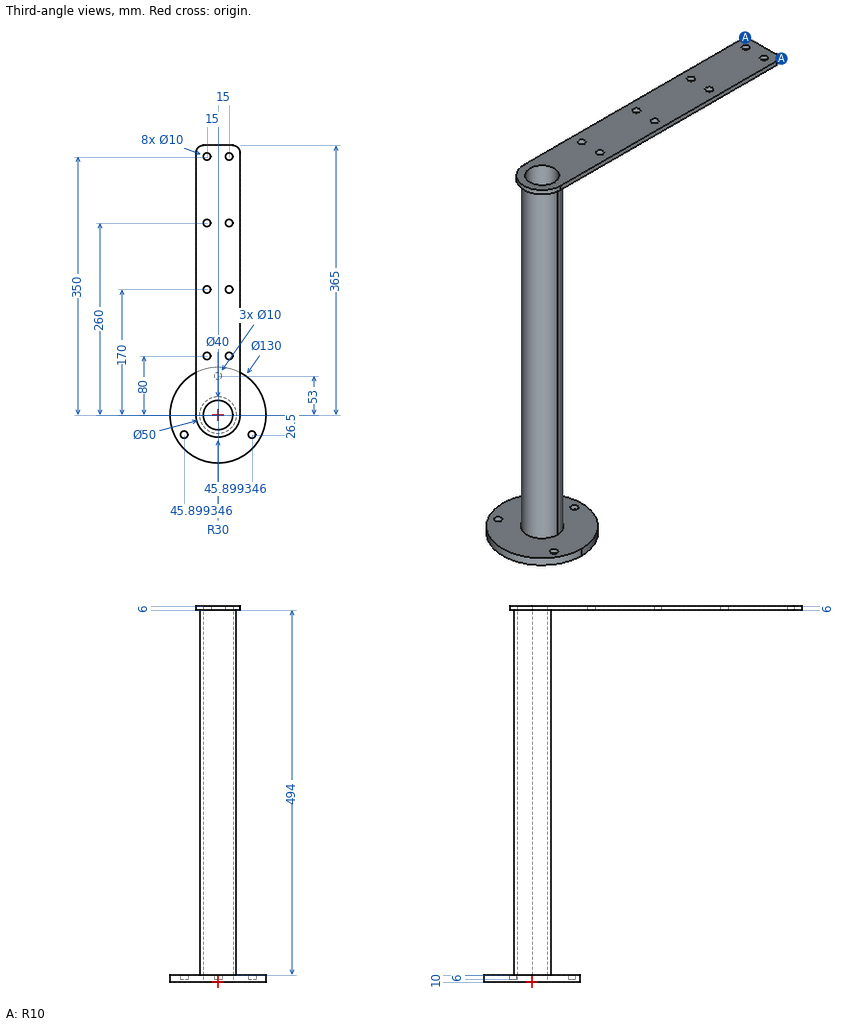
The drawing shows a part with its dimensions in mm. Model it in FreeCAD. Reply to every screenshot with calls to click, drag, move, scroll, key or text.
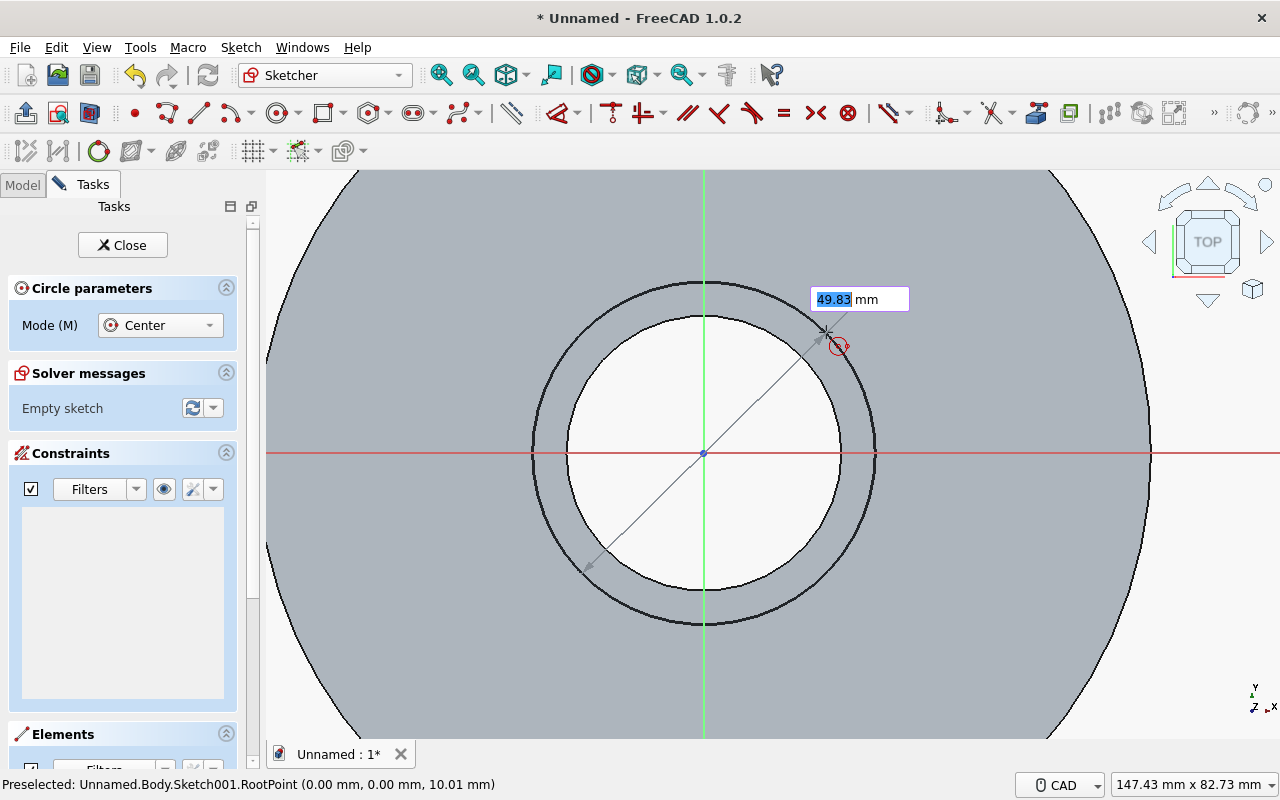
text(50)
key(Return)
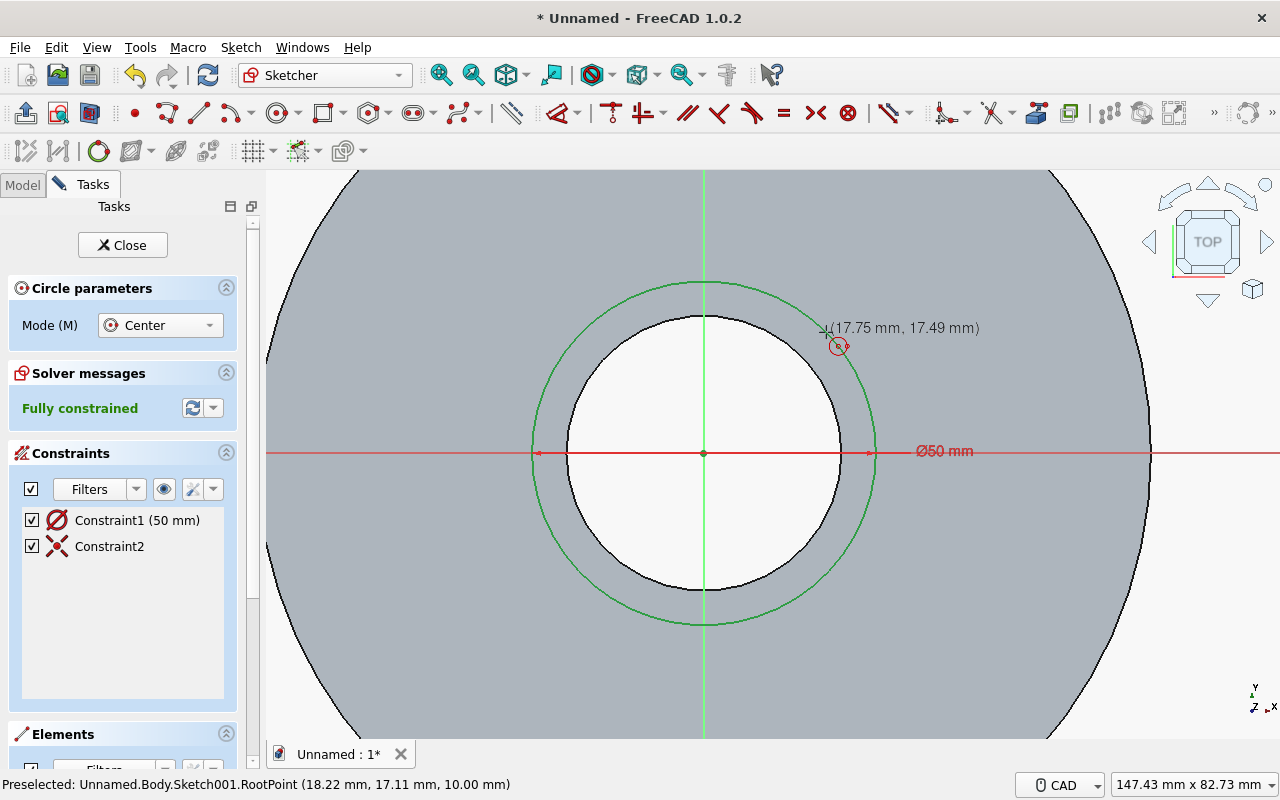
click(704, 453)
move(801, 356)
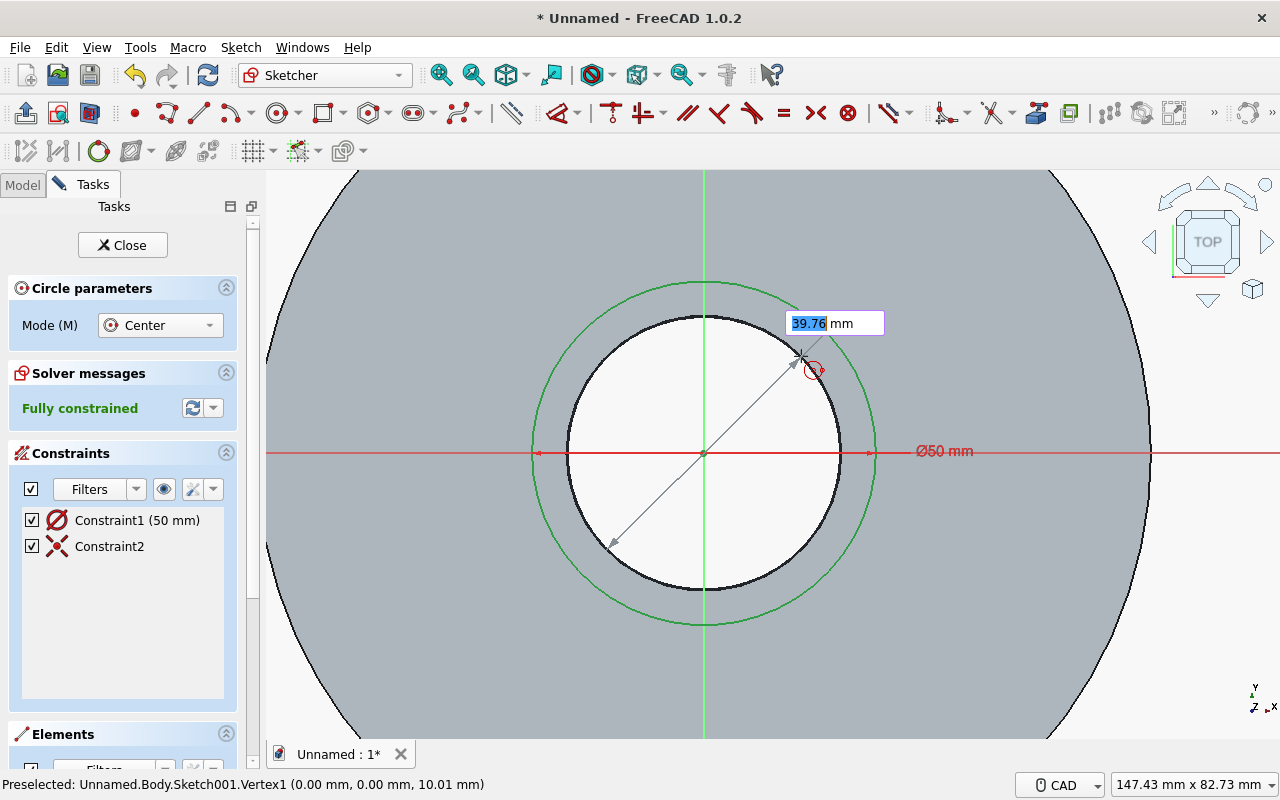
text(40)
key(Return)
key(Escape)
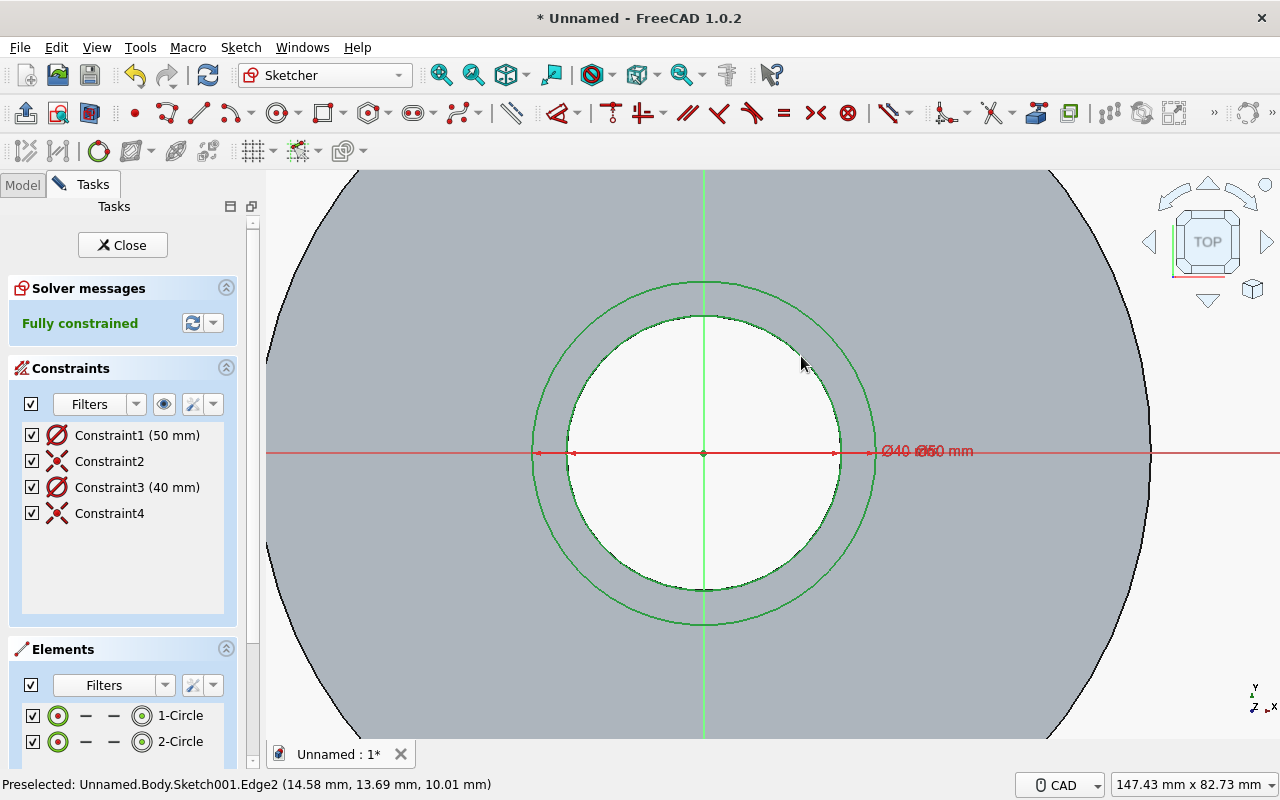
click(123, 245)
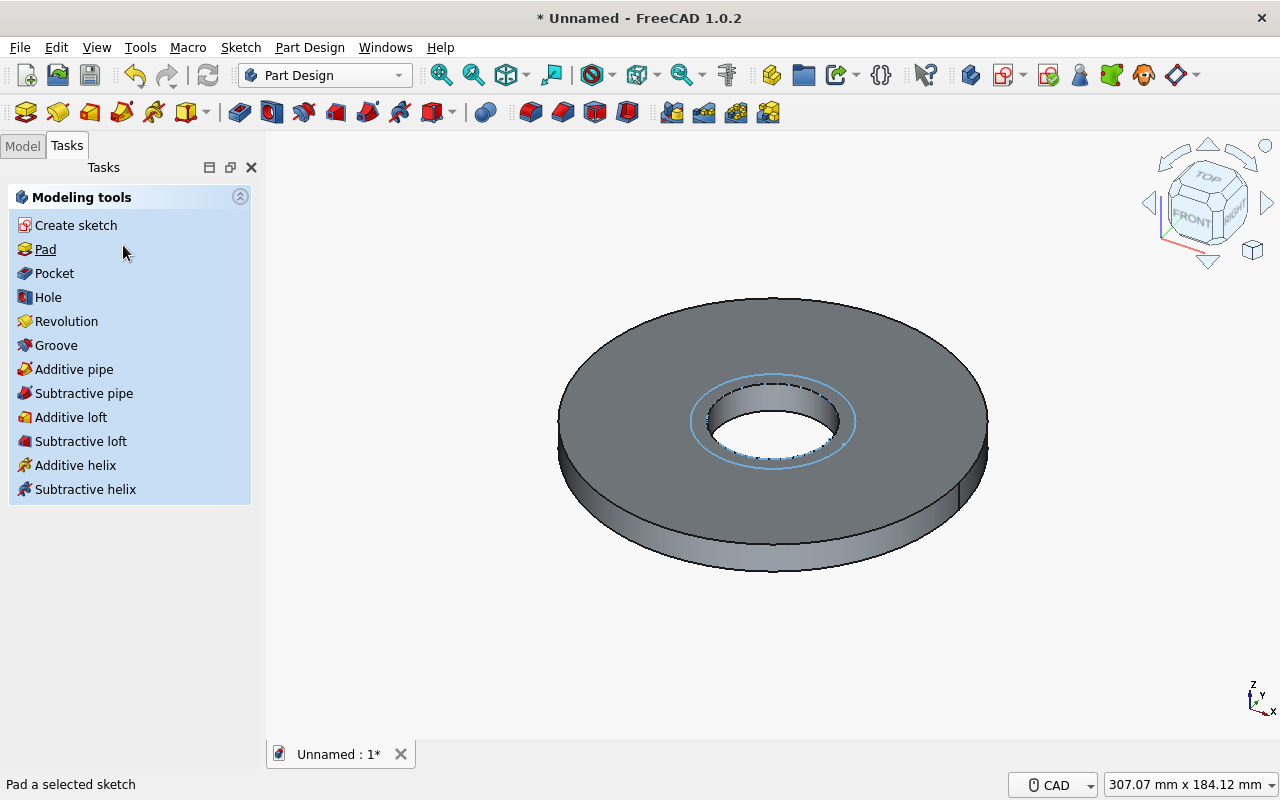
click(26, 112)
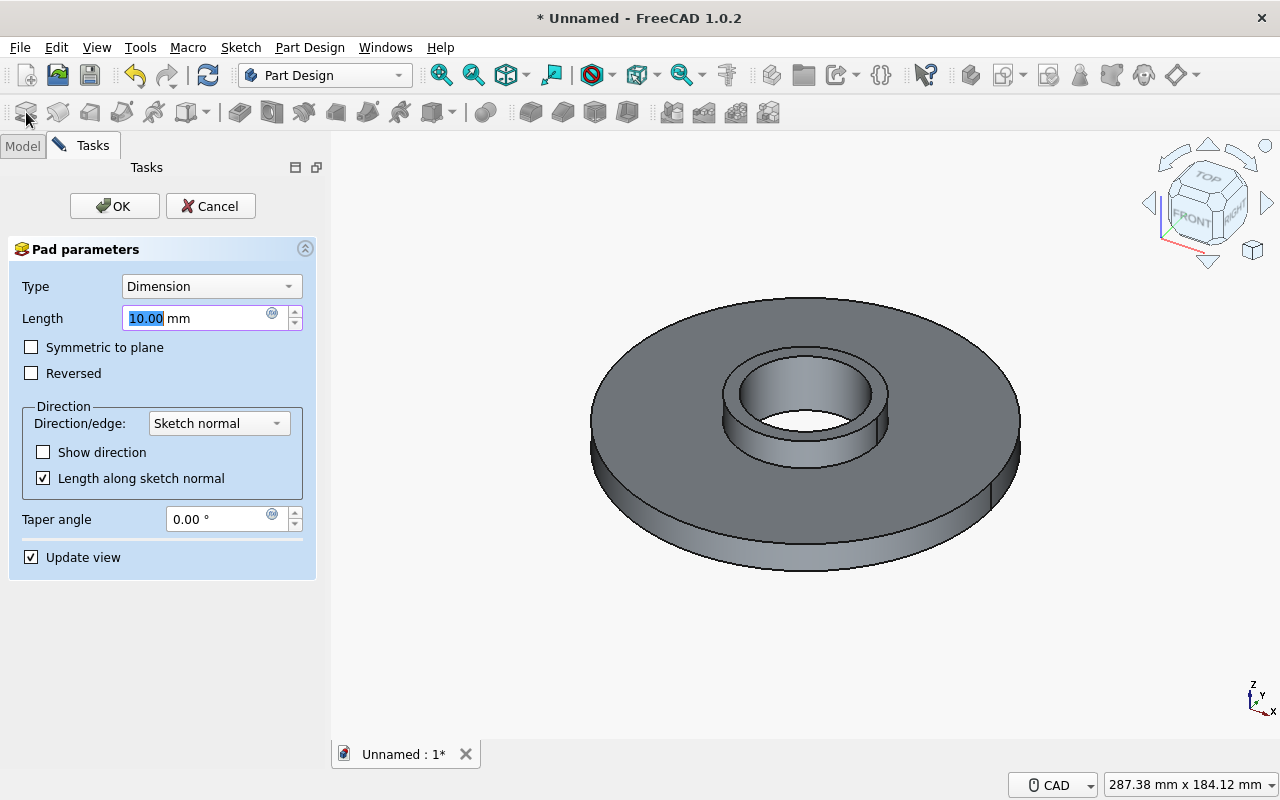
text(494)
key(Tab)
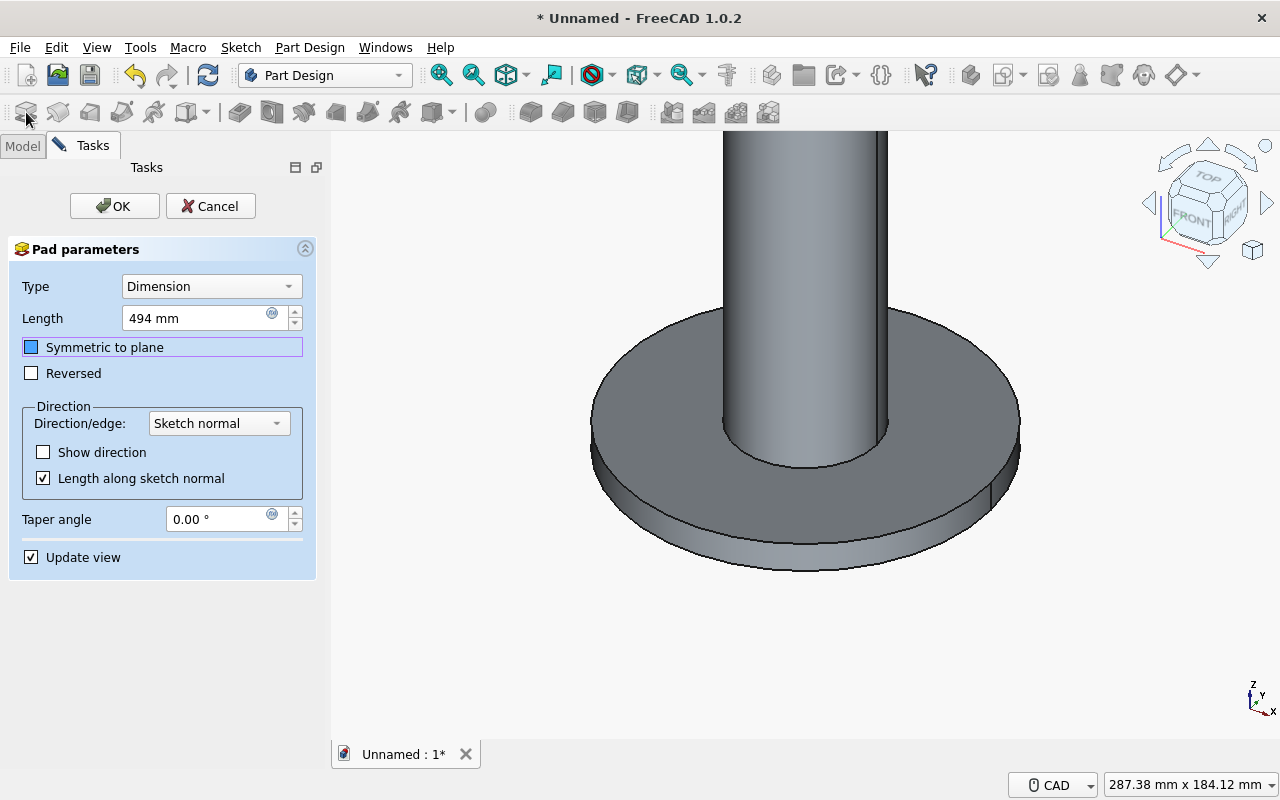
click(115, 206)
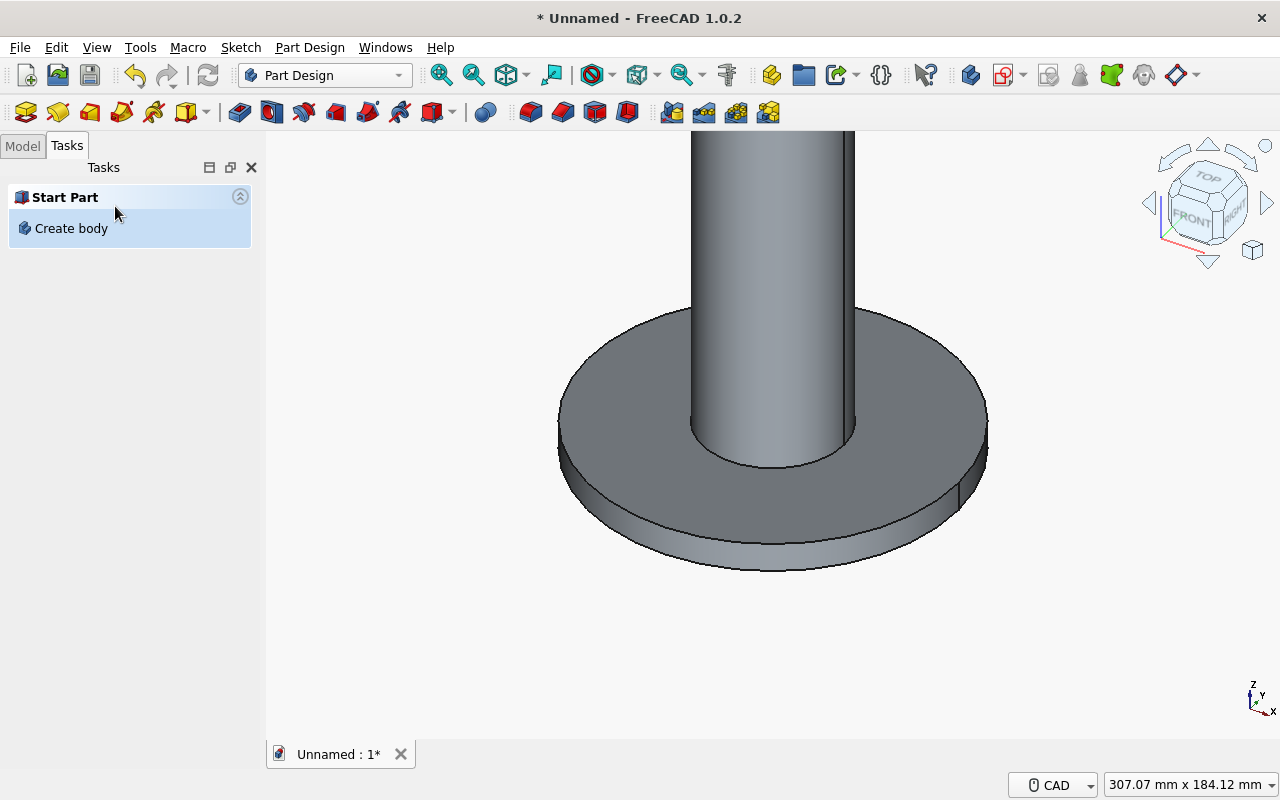
click(442, 76)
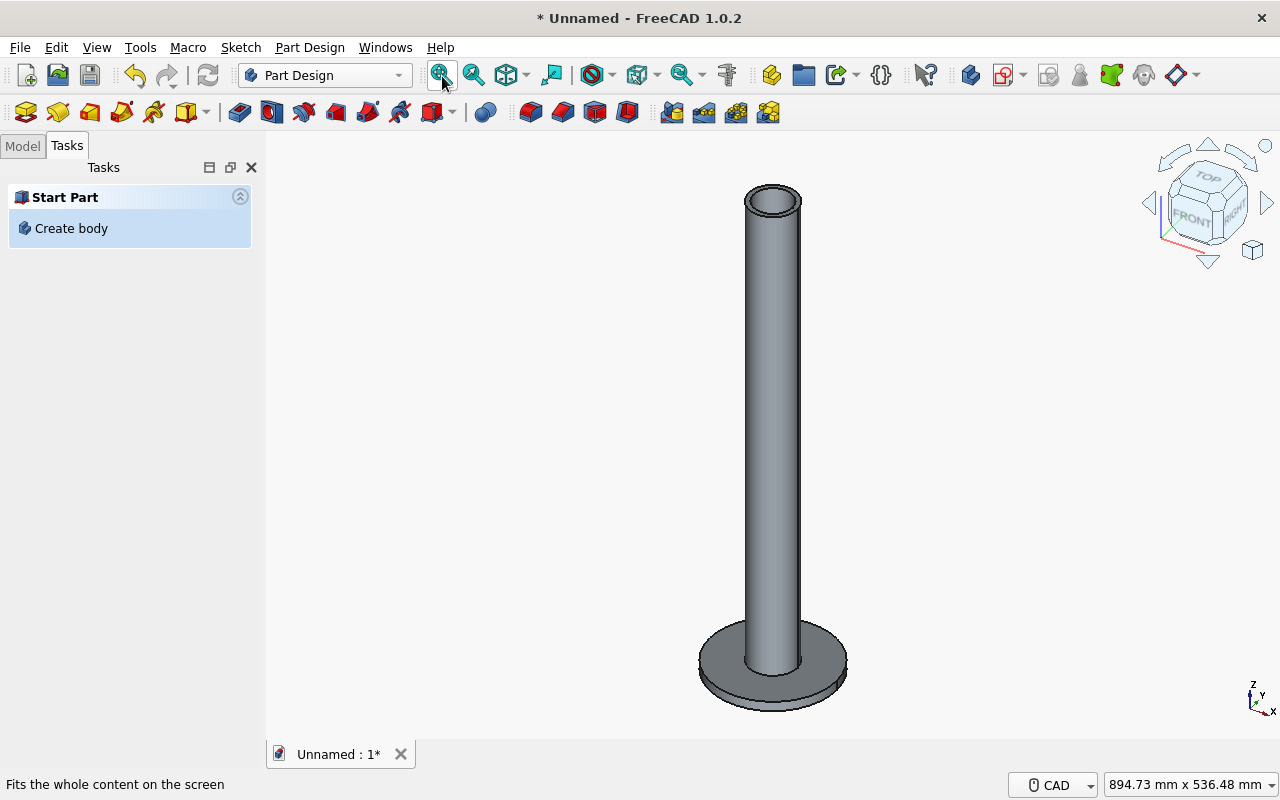
scroll(748, 197, up, 8)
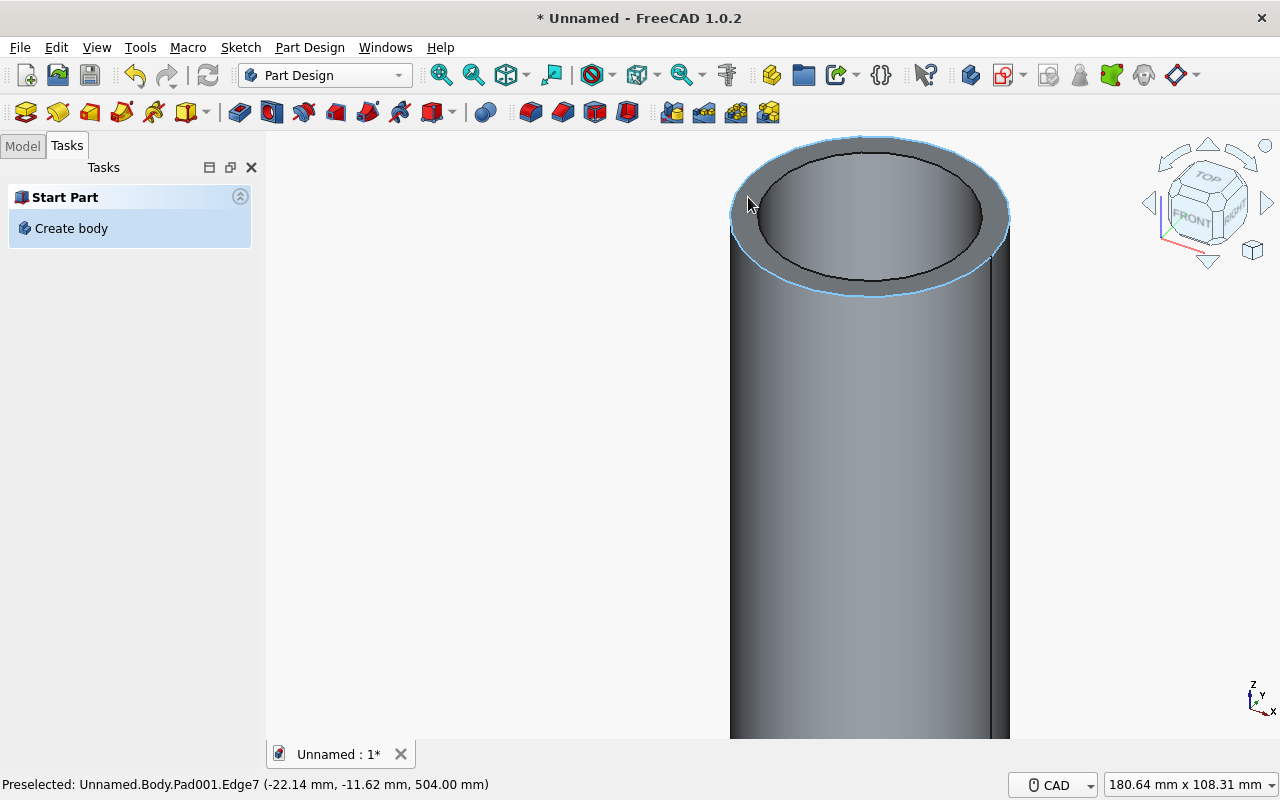
click(746, 201)